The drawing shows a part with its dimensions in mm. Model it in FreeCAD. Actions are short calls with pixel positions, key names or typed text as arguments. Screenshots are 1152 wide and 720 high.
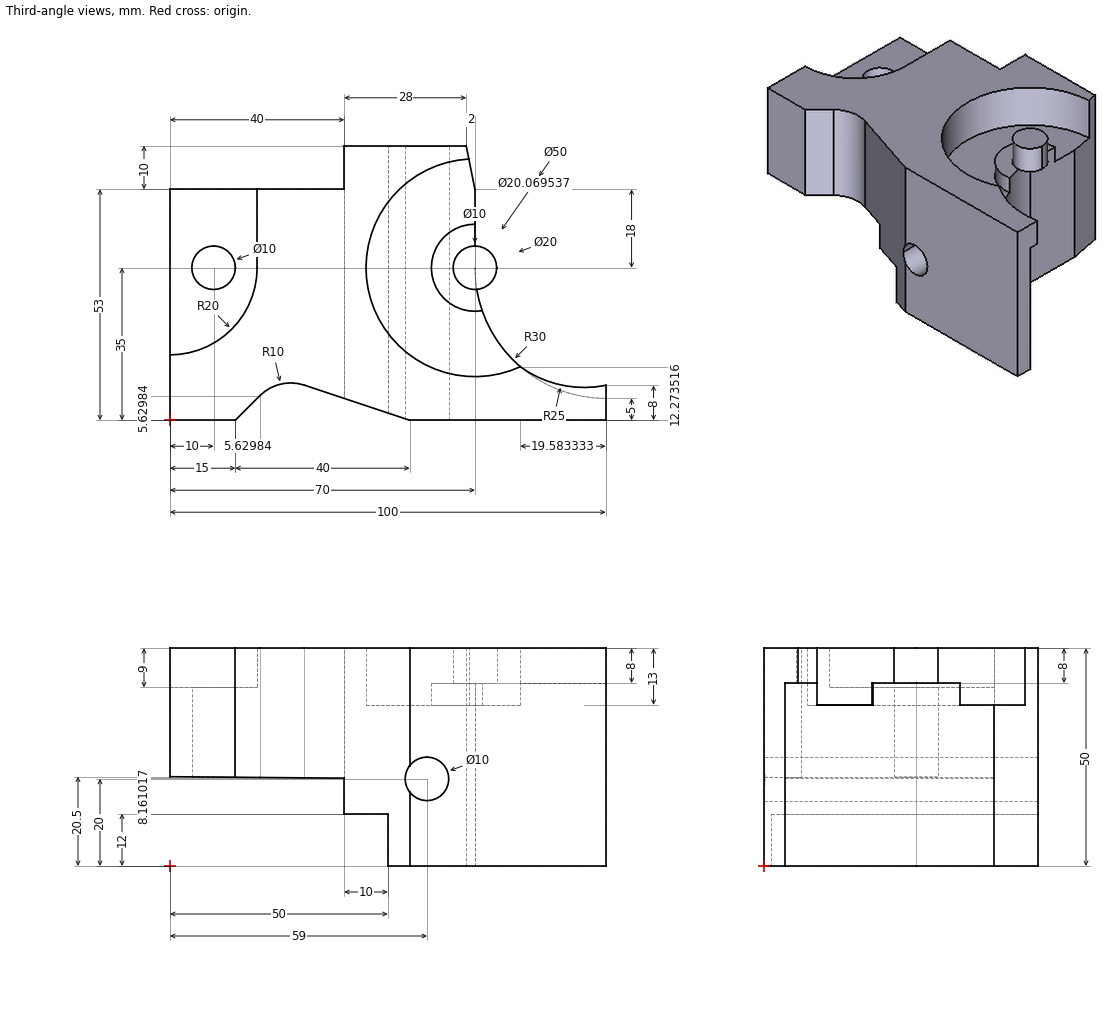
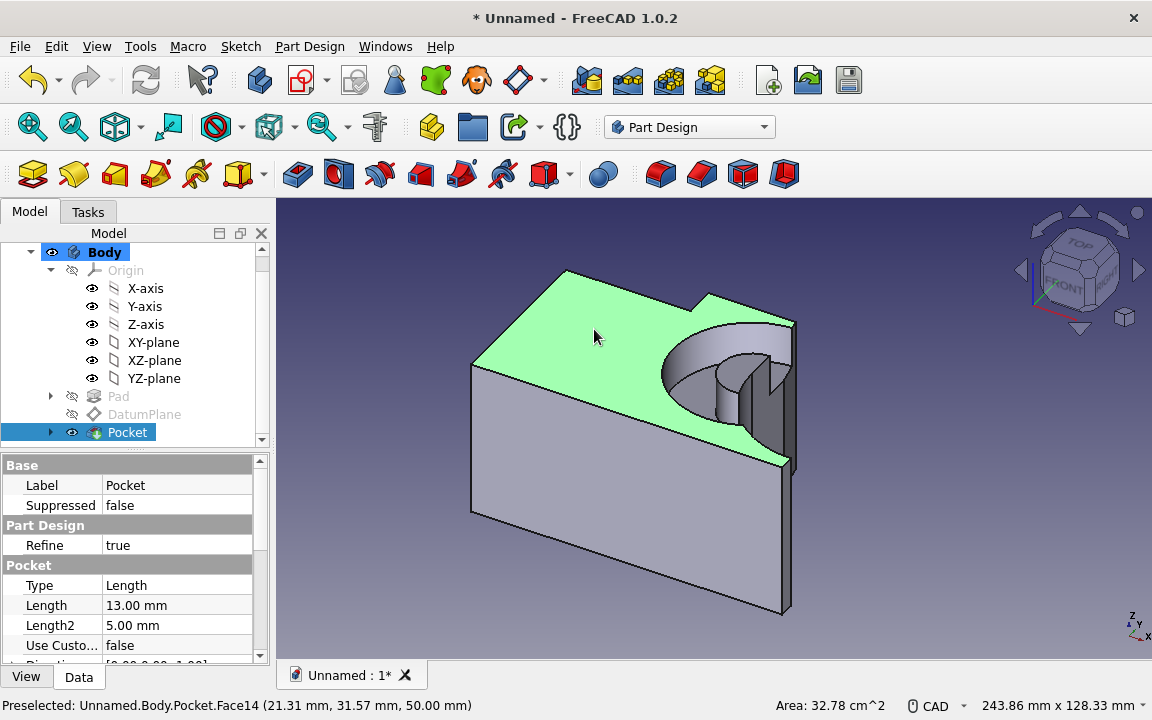
click(300, 80)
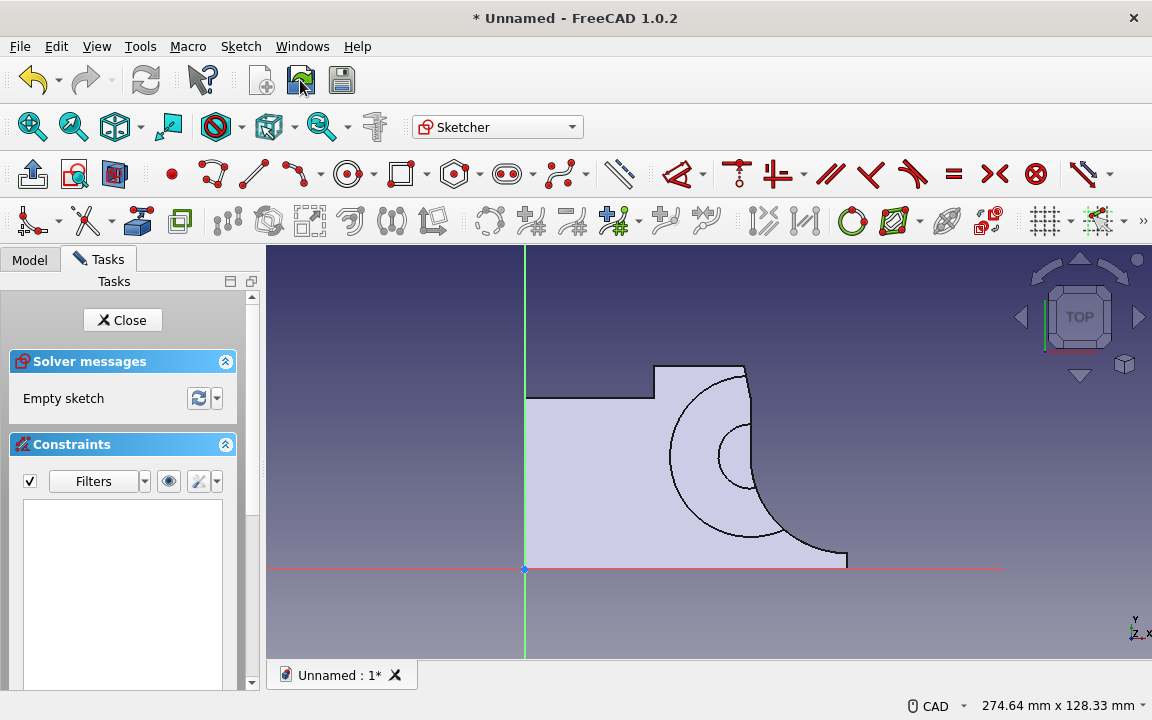
scroll(787, 458, up, 7)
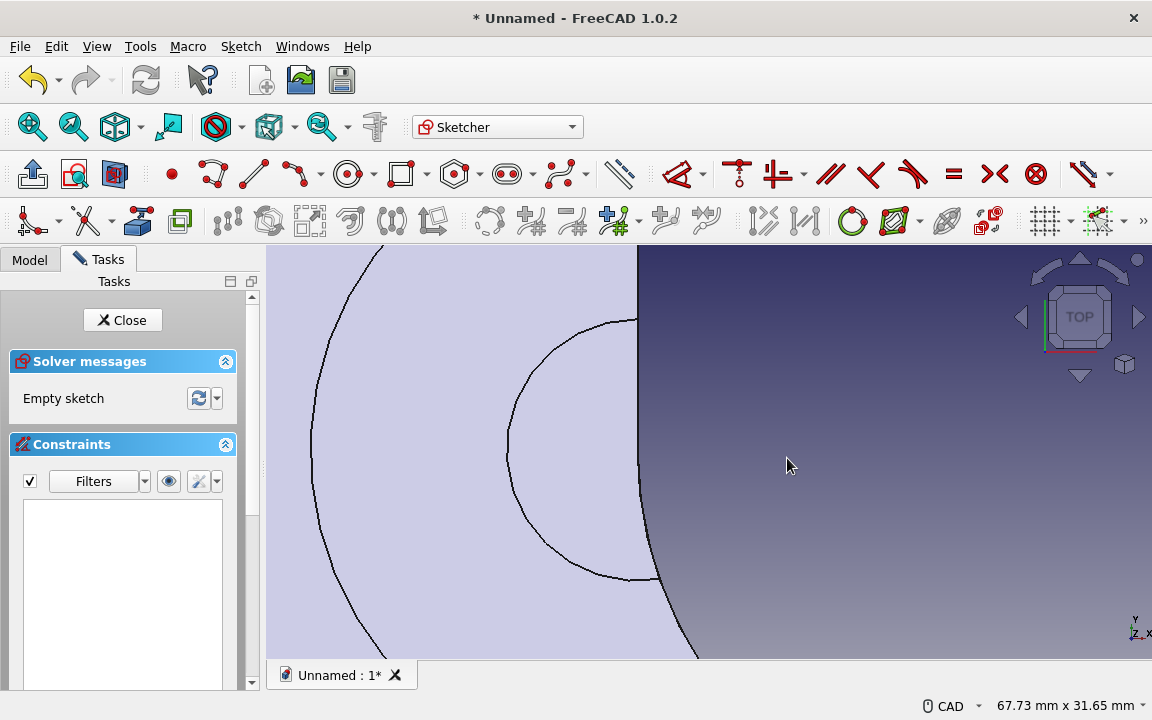
click(348, 174)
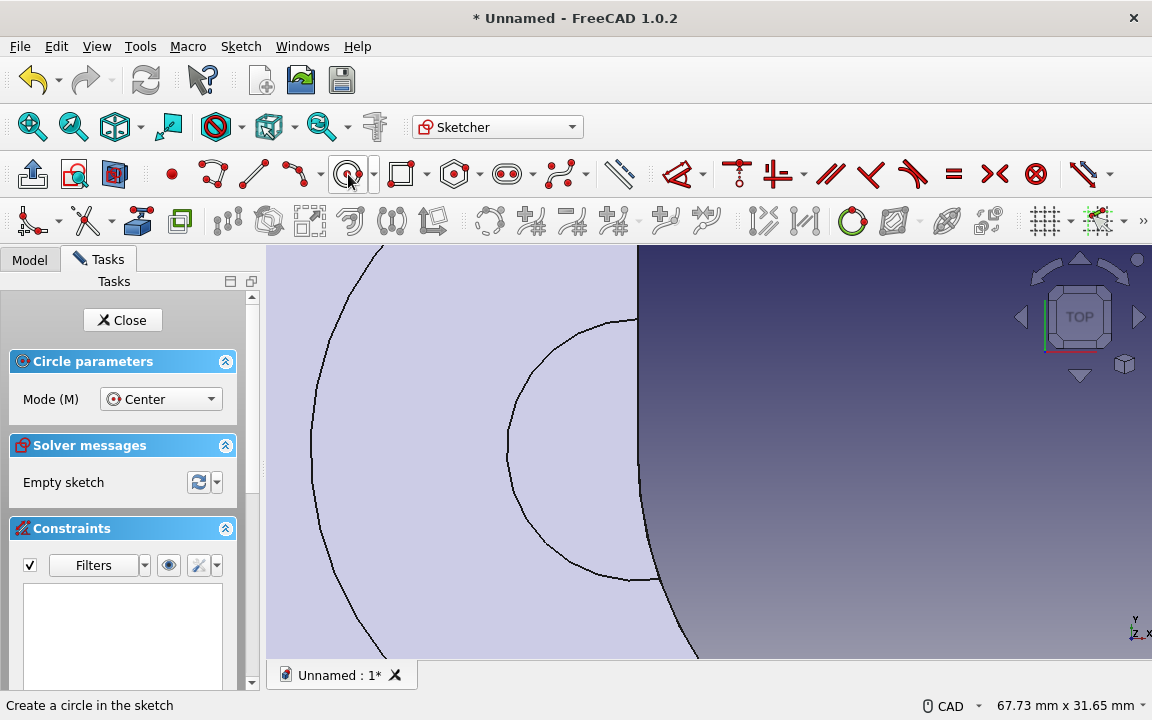
click(638, 450)
click(730, 357)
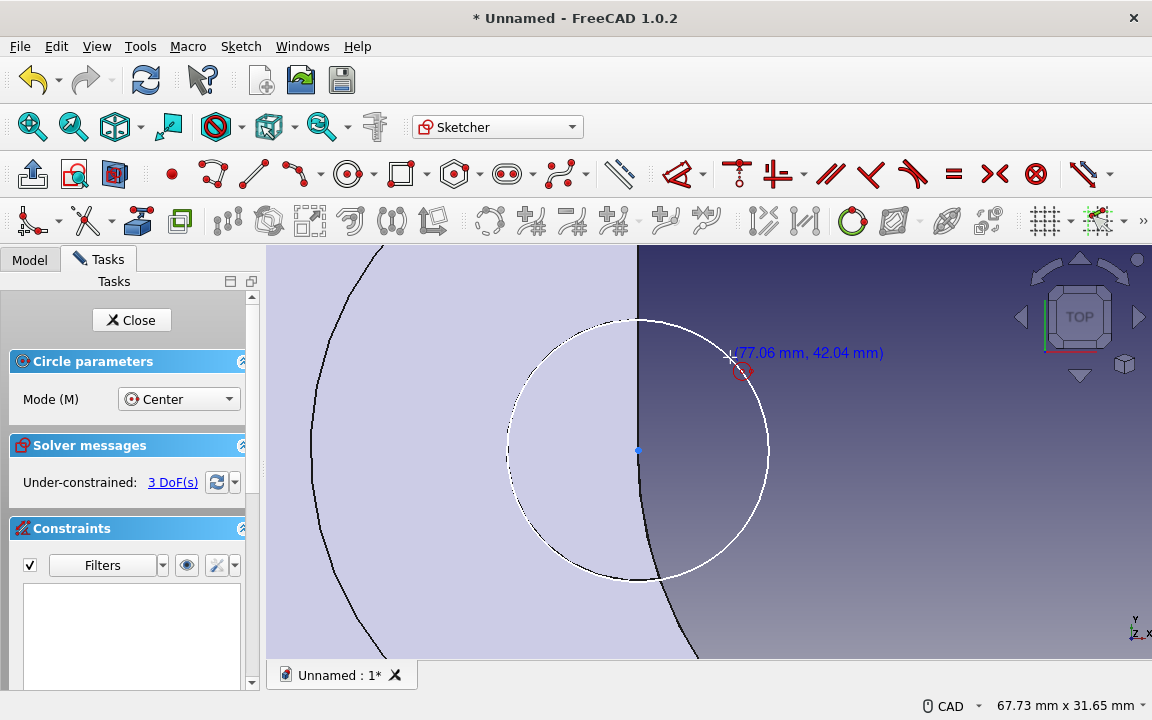
click(638, 451)
click(684, 404)
key(Escape)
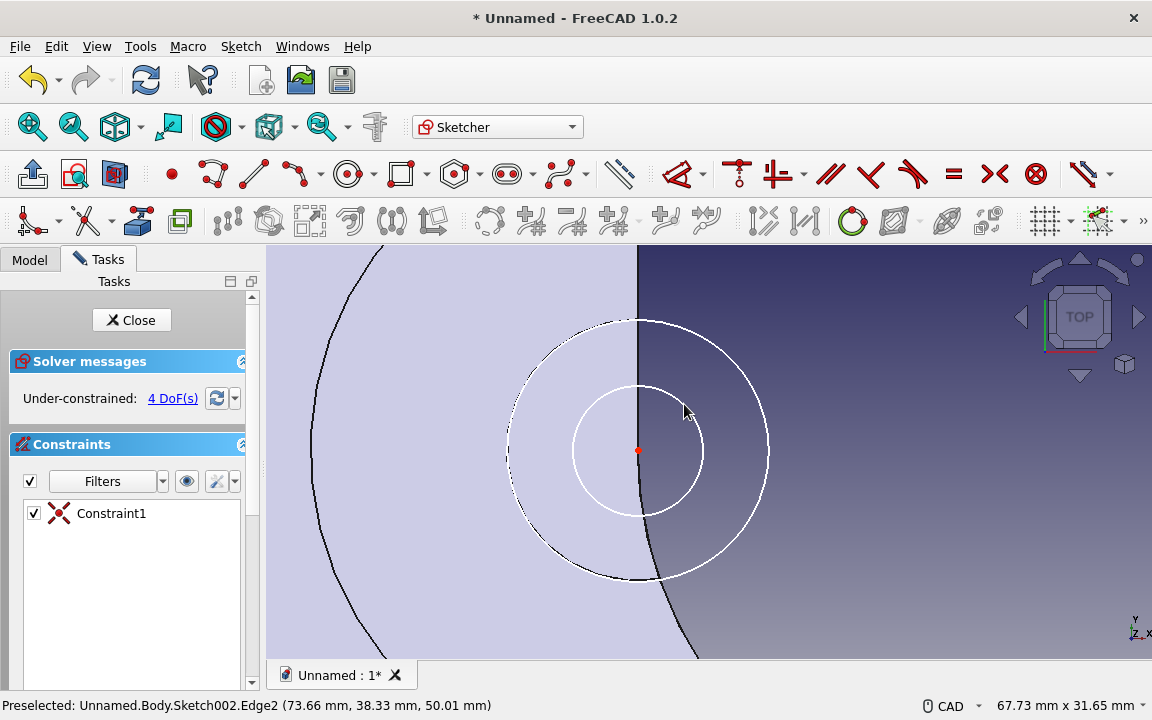
key(d)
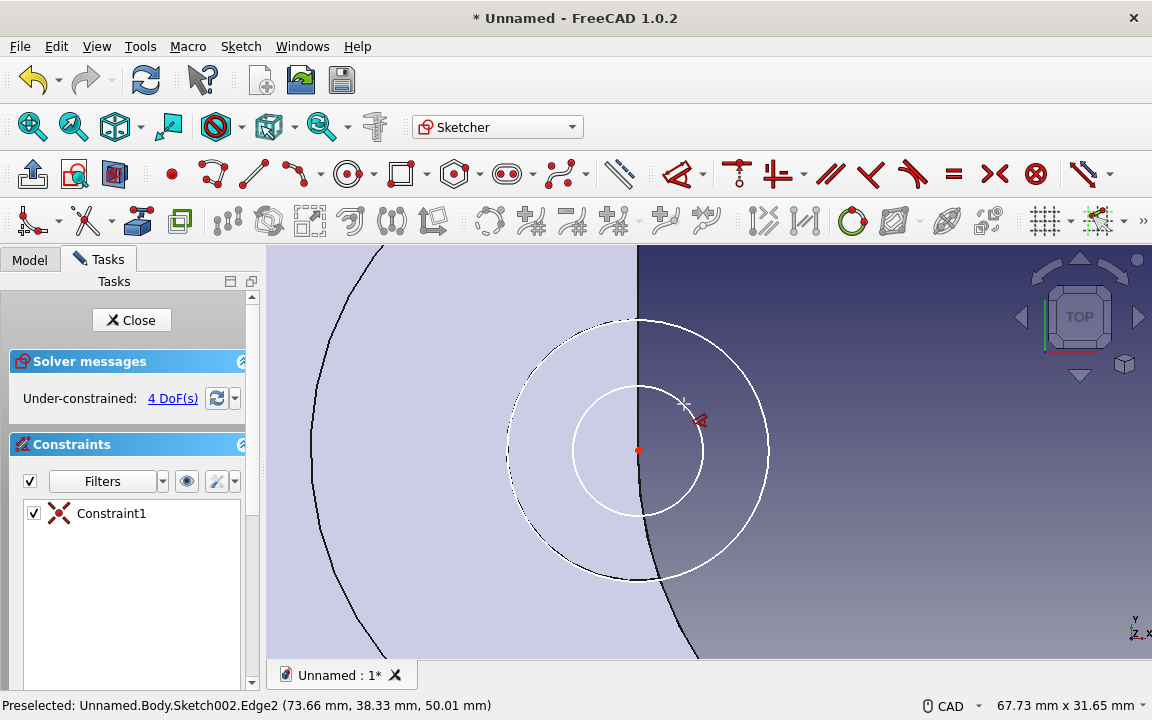
click(730, 358)
click(753, 335)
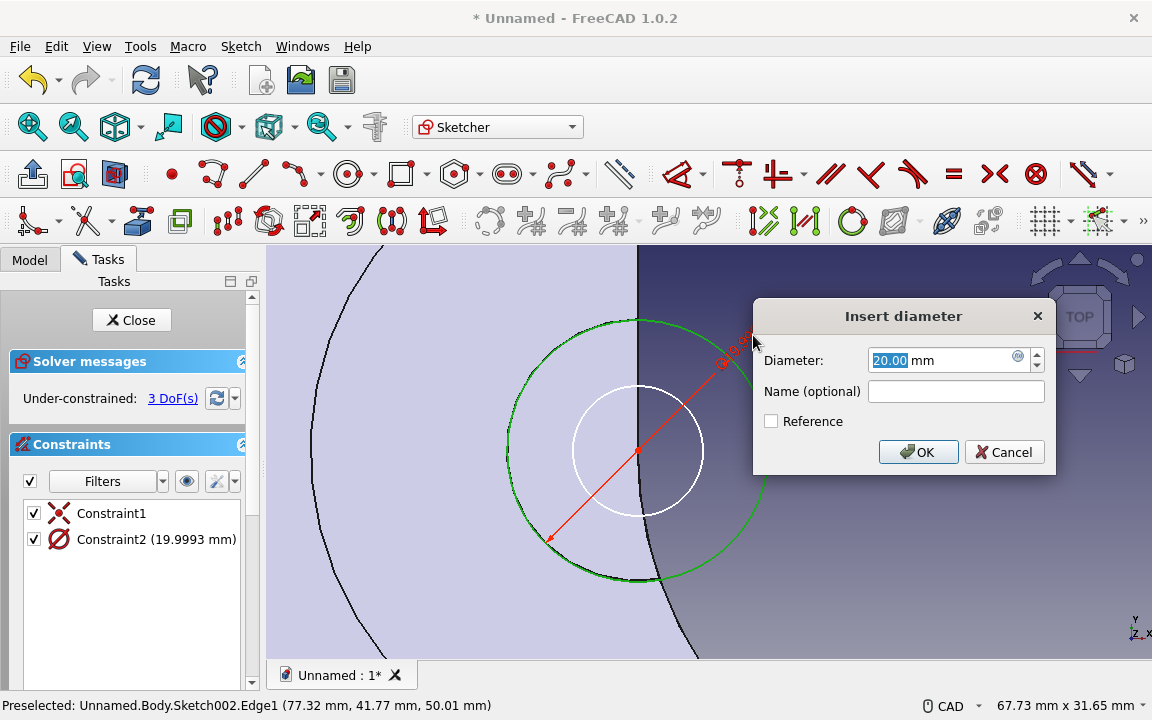
text(20.069537)
key(Return)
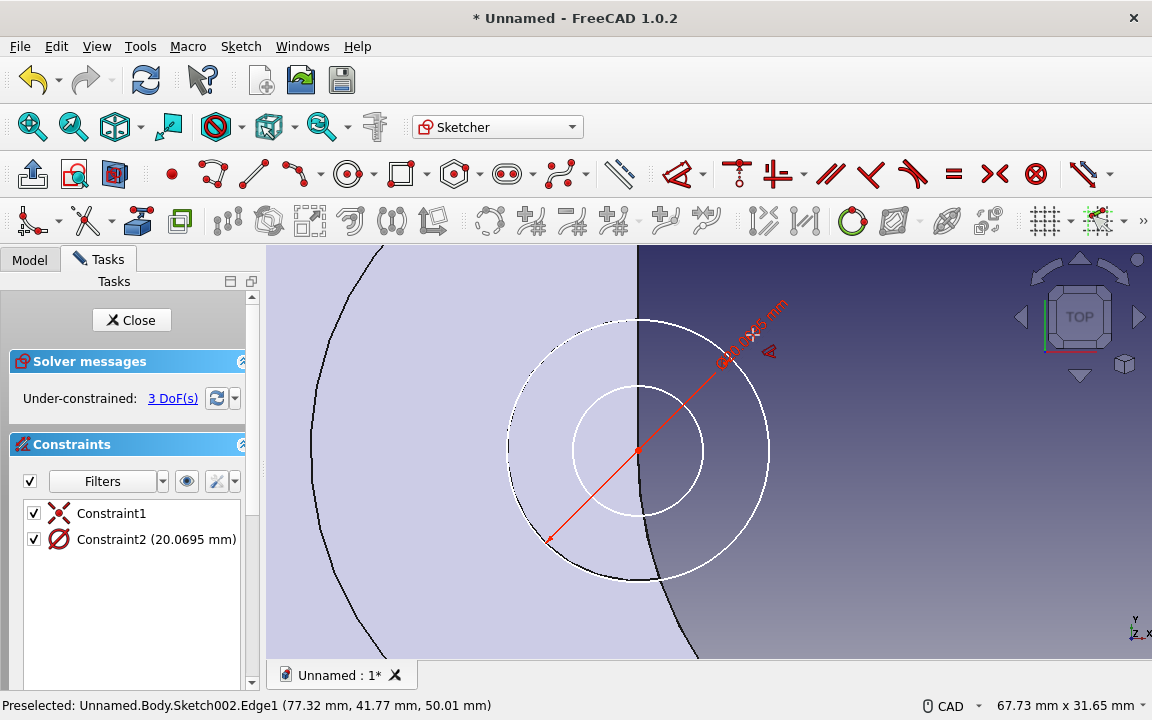
click(684, 405)
click(707, 382)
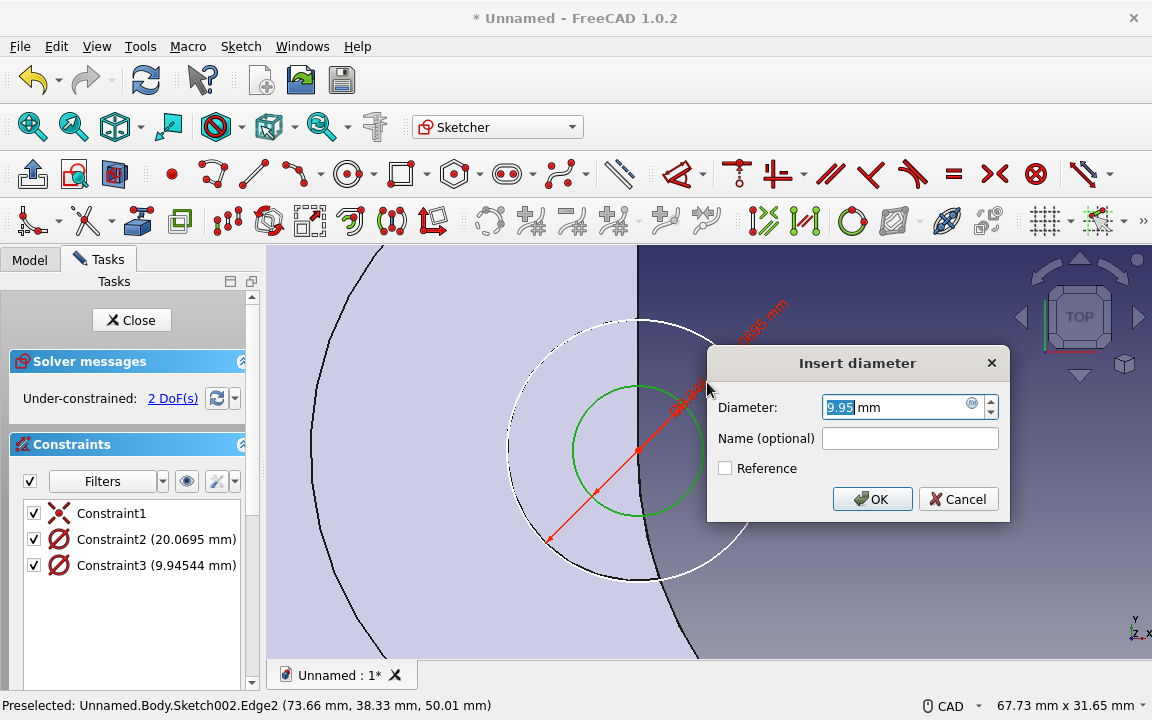
text(10)
key(Return)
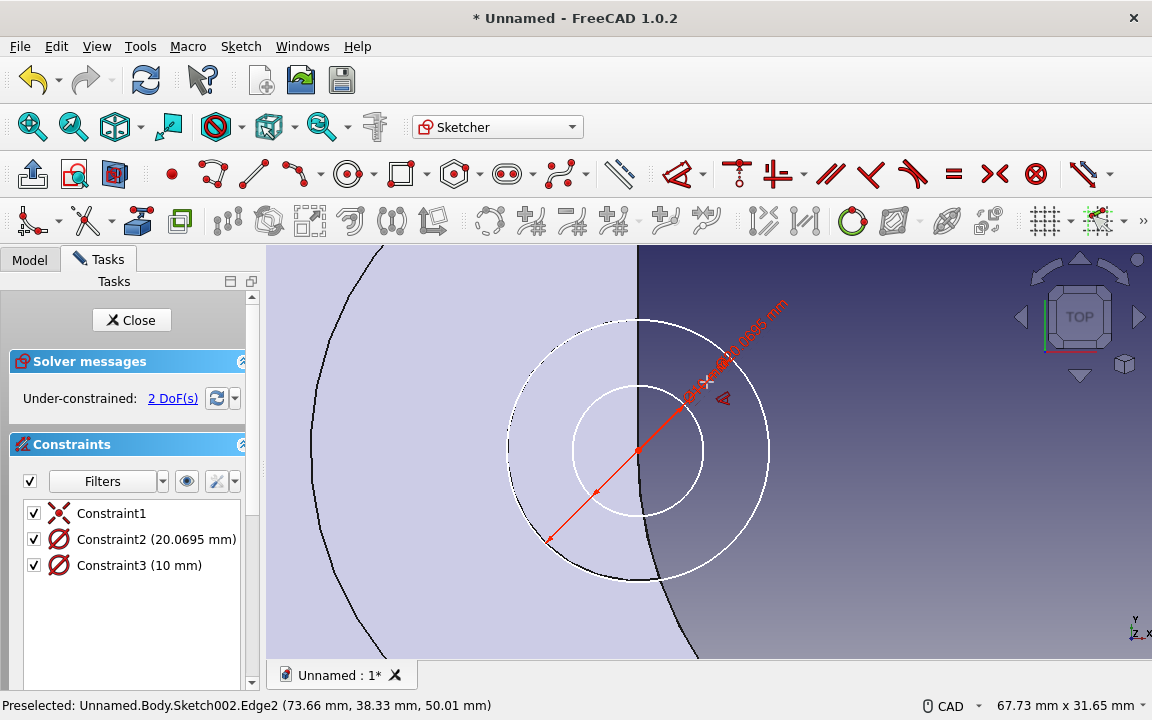
click(638, 451)
click(466, 417)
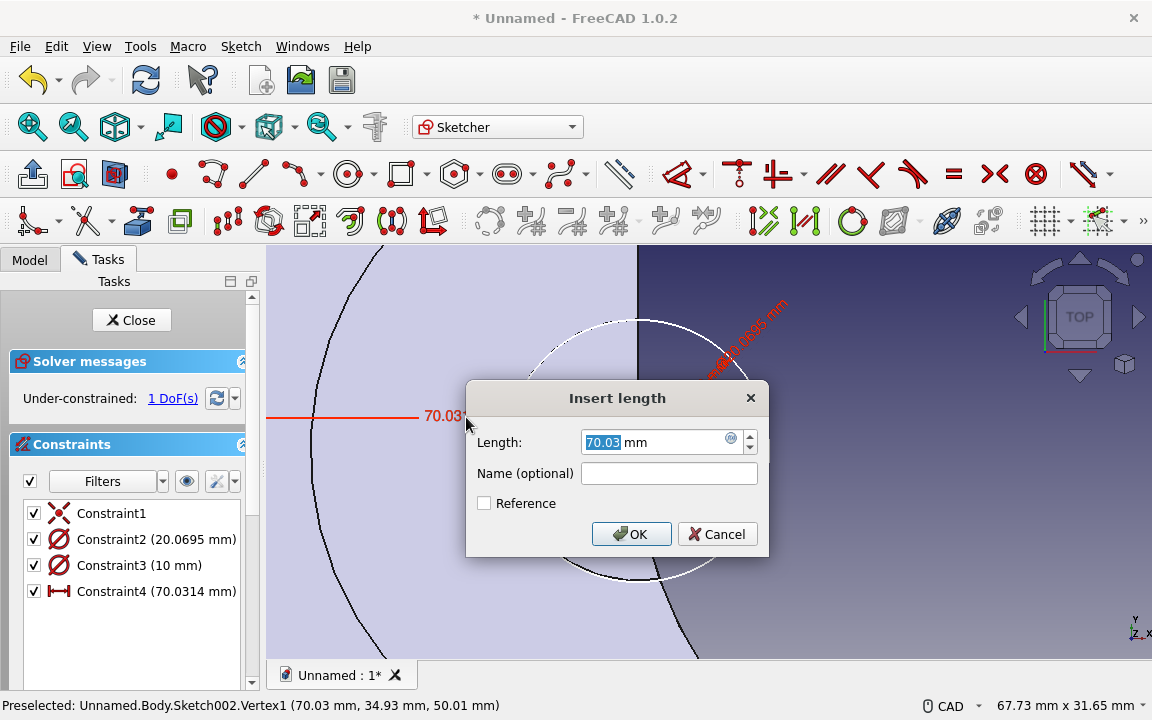
text(70)
key(Return)